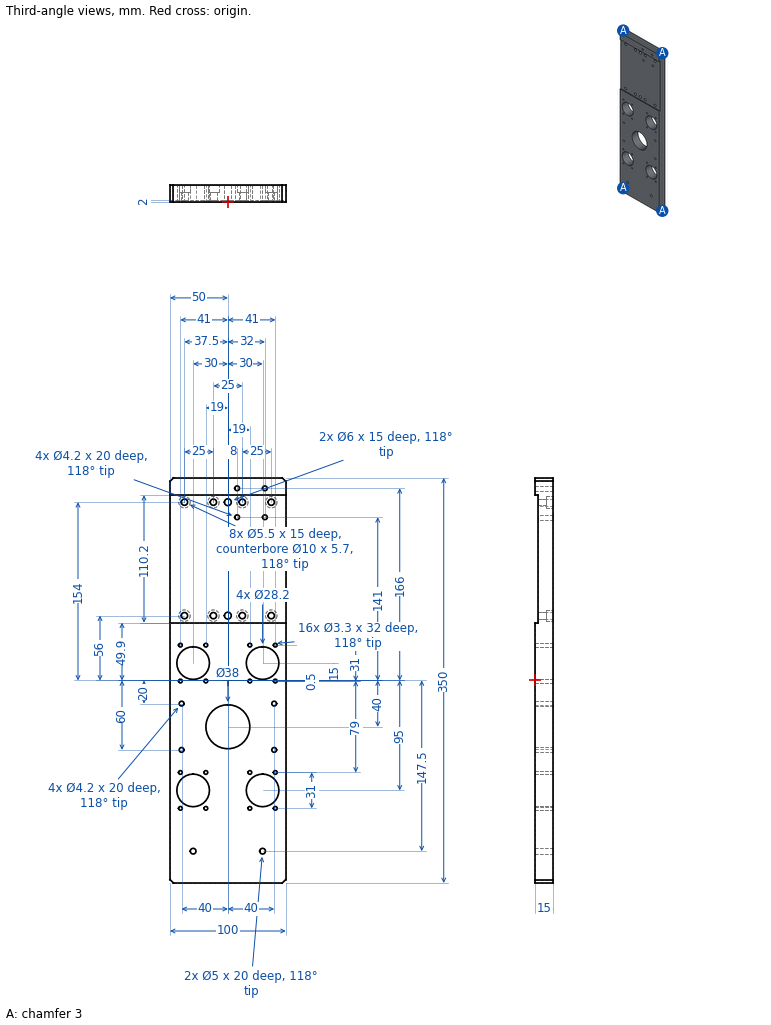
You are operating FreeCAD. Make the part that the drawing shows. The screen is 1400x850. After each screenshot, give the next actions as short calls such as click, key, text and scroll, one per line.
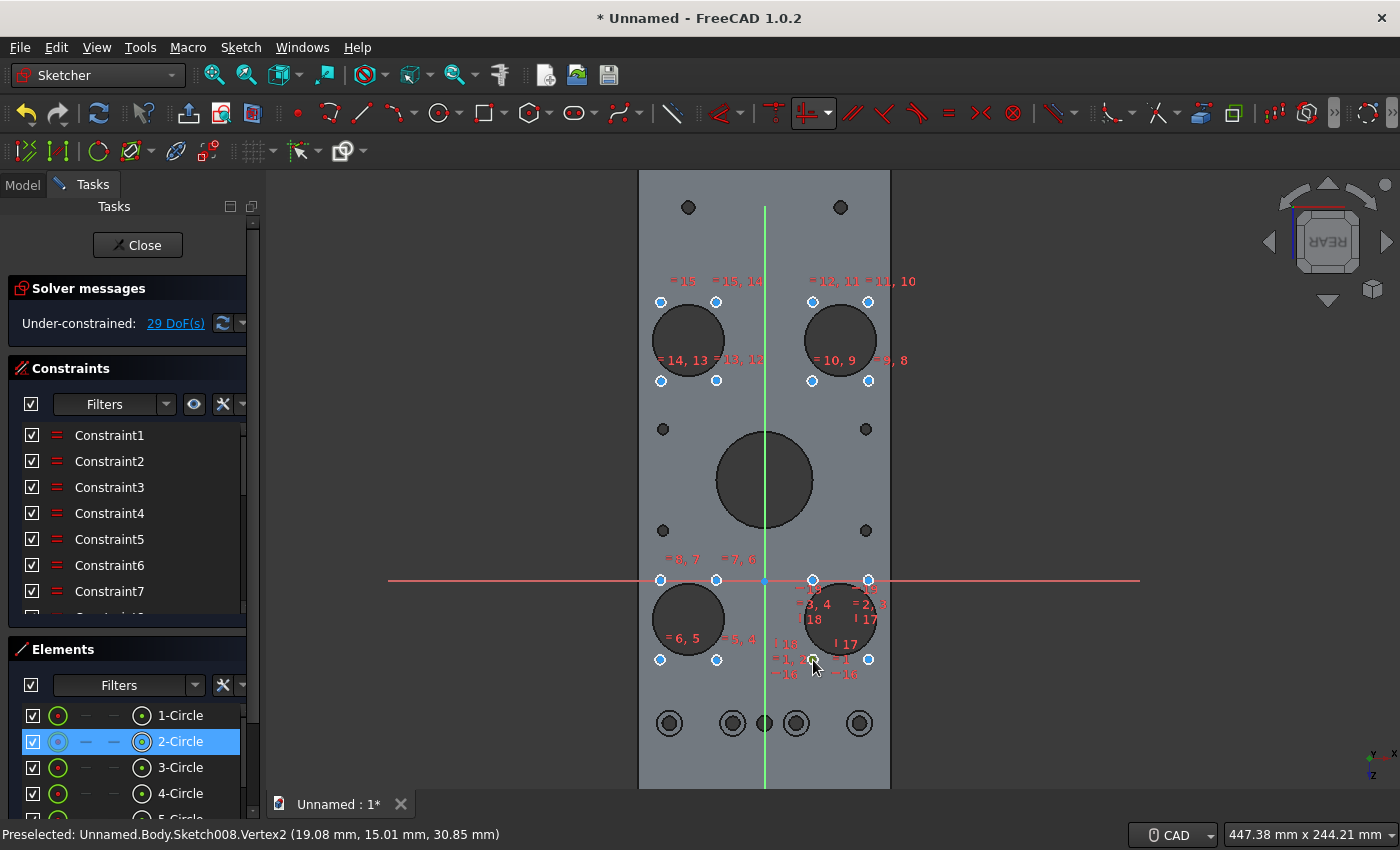
click(717, 660)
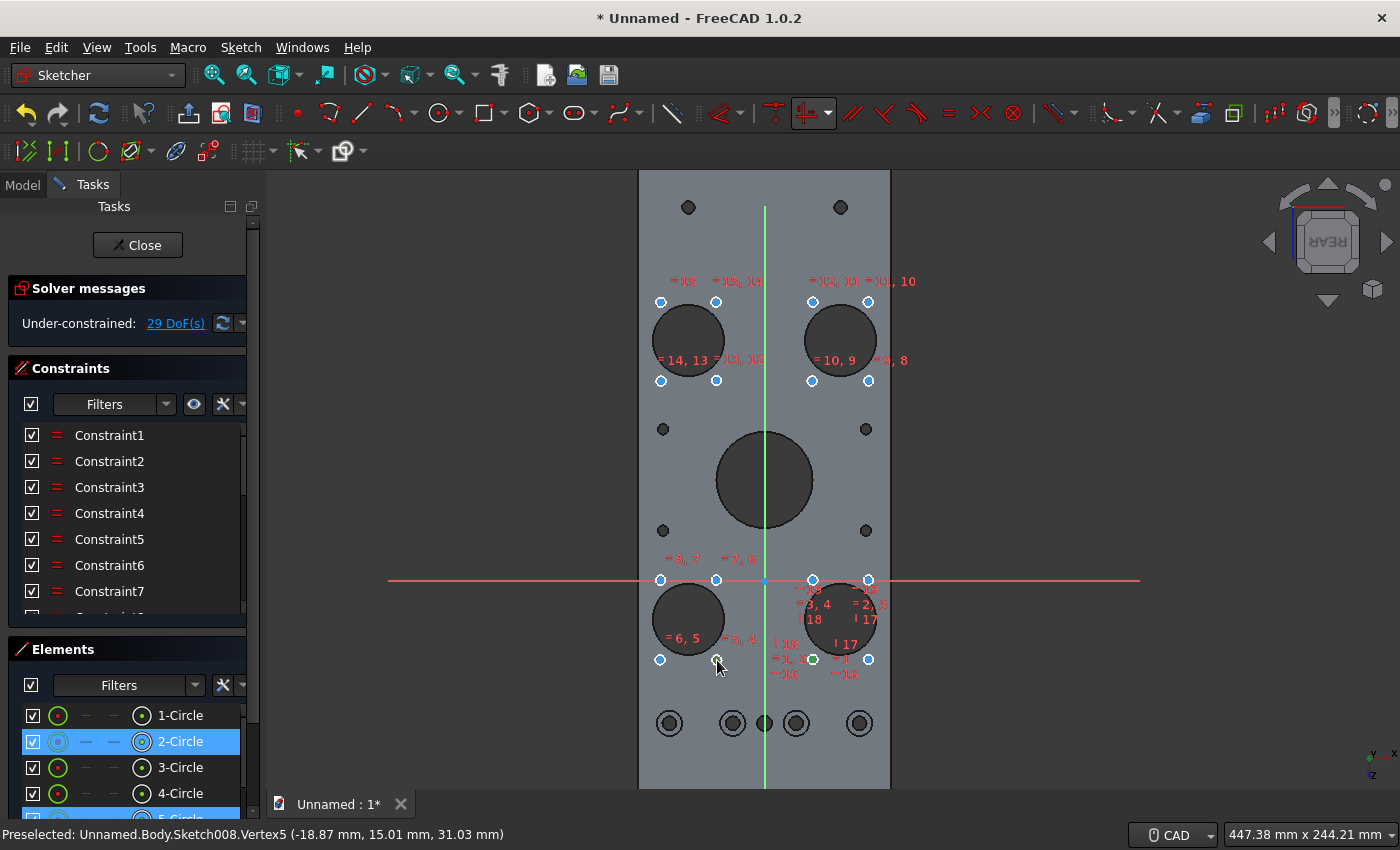
key(h)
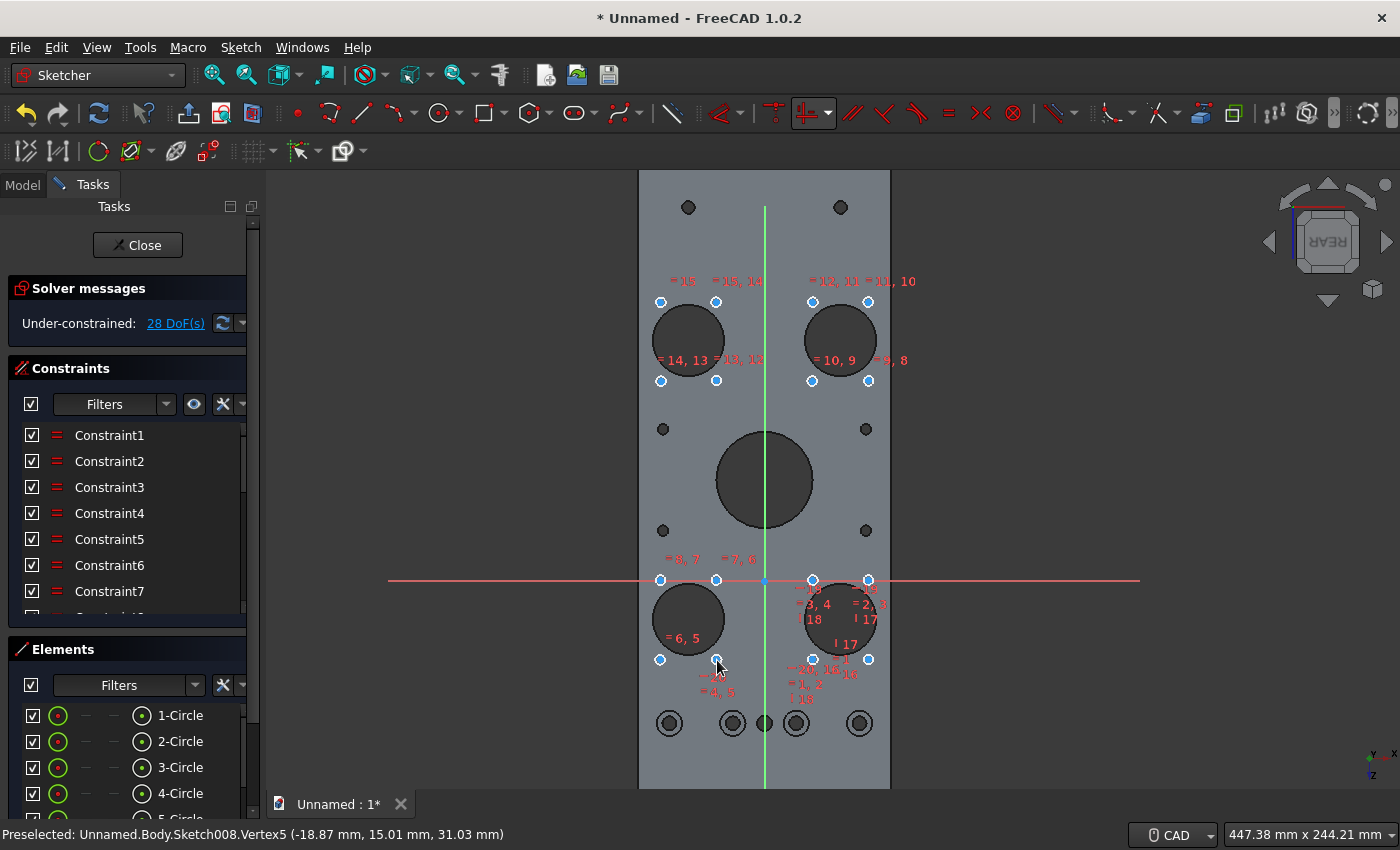
click(717, 660)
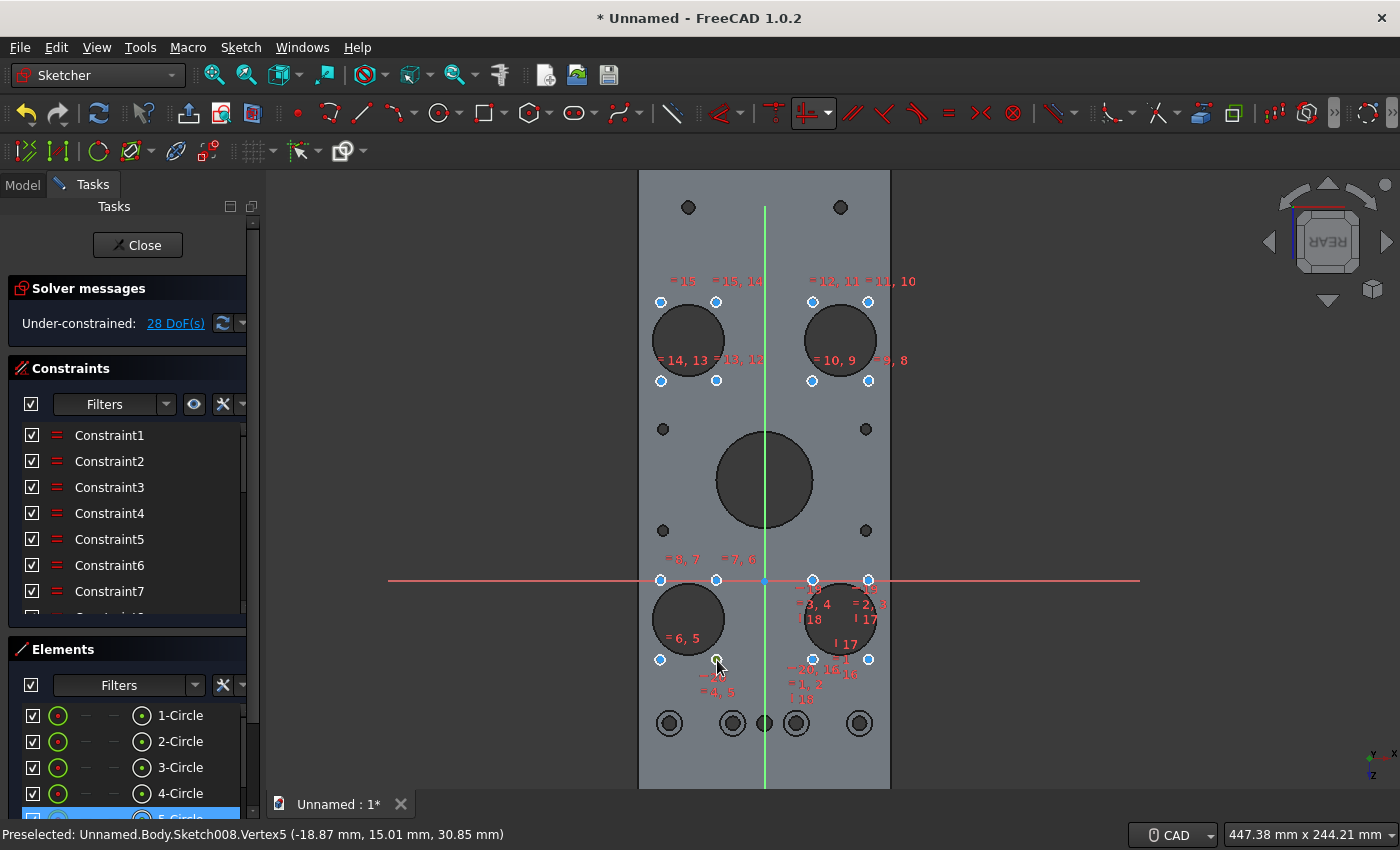
click(660, 660)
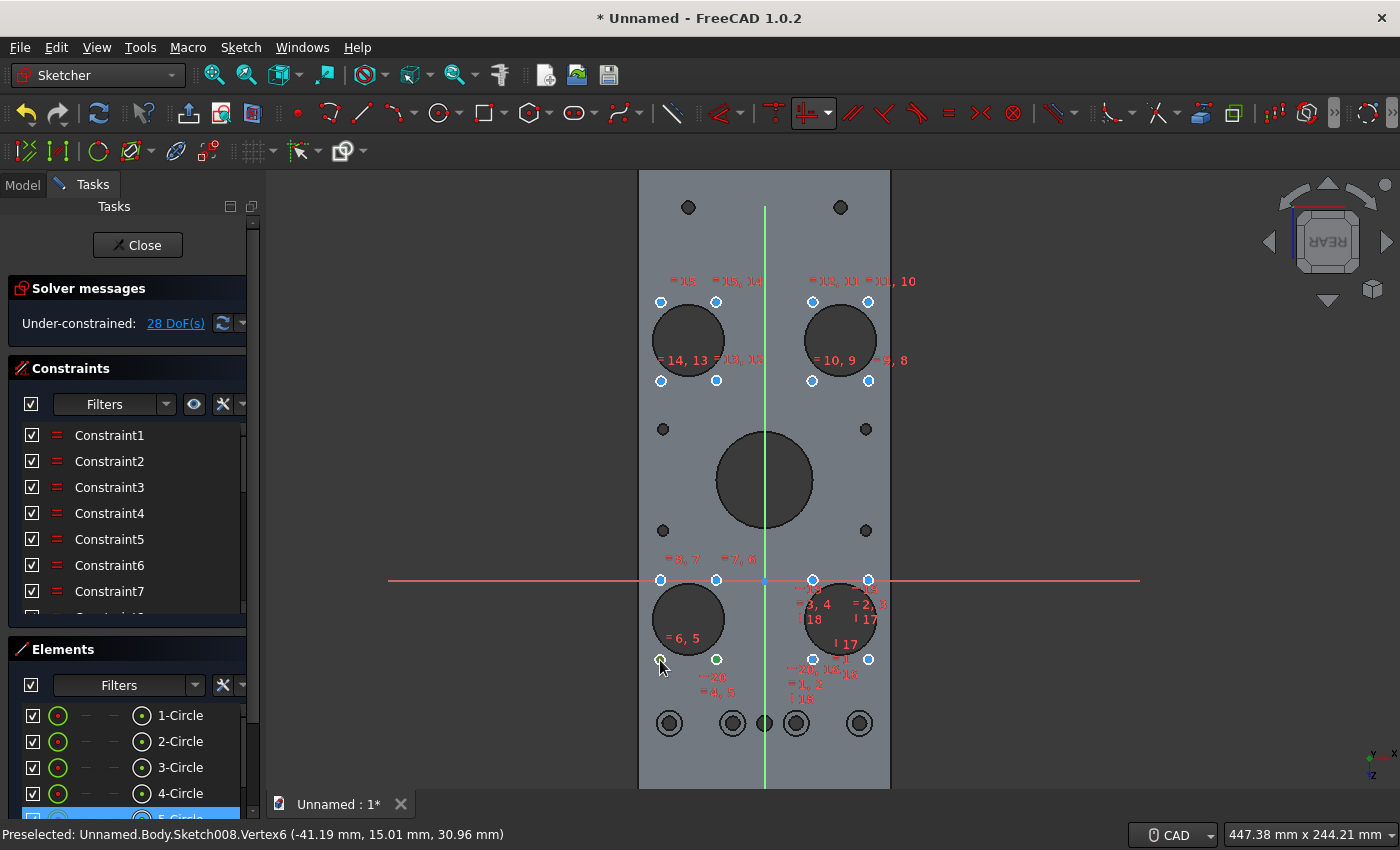
click(830, 114)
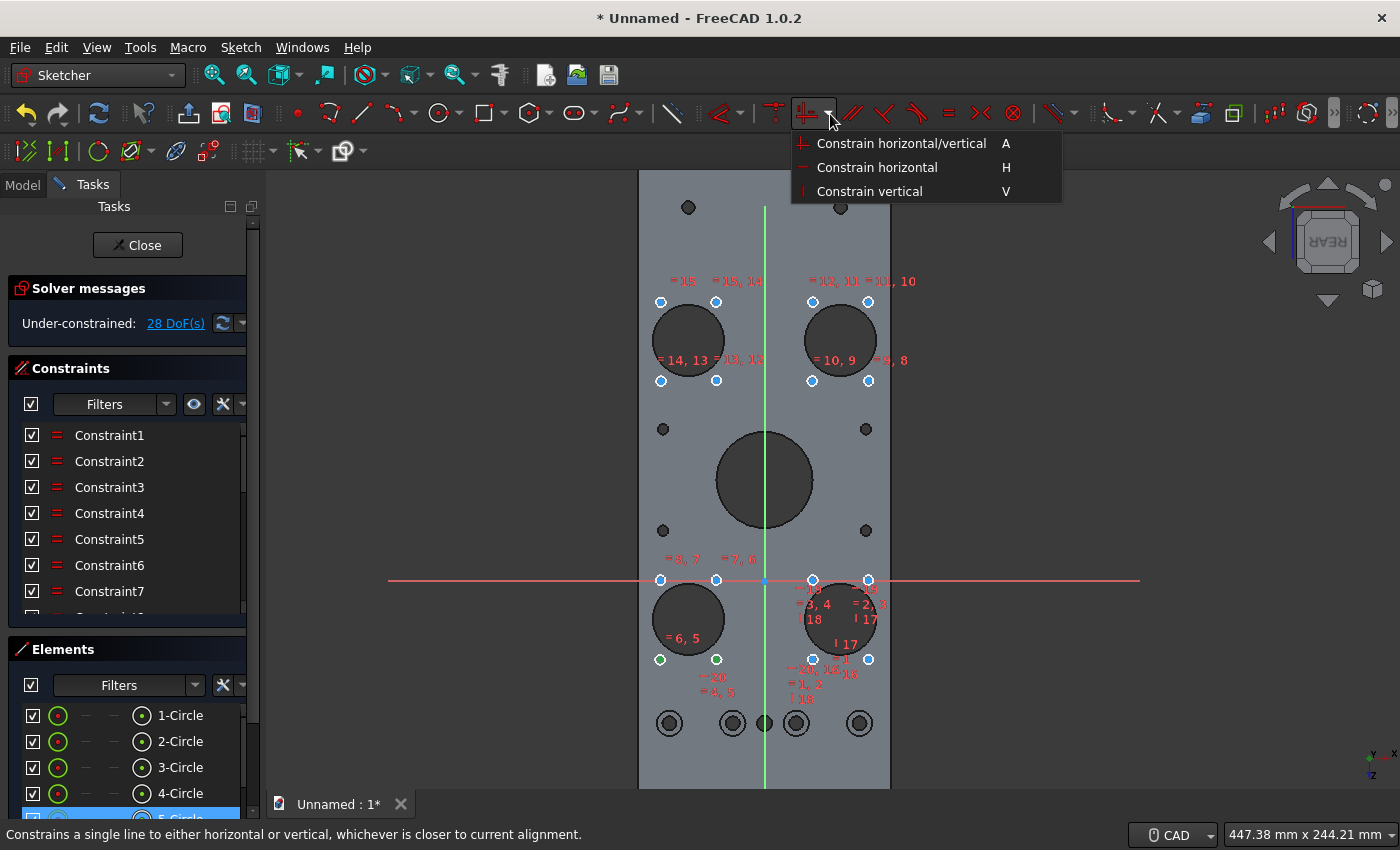
click(927, 167)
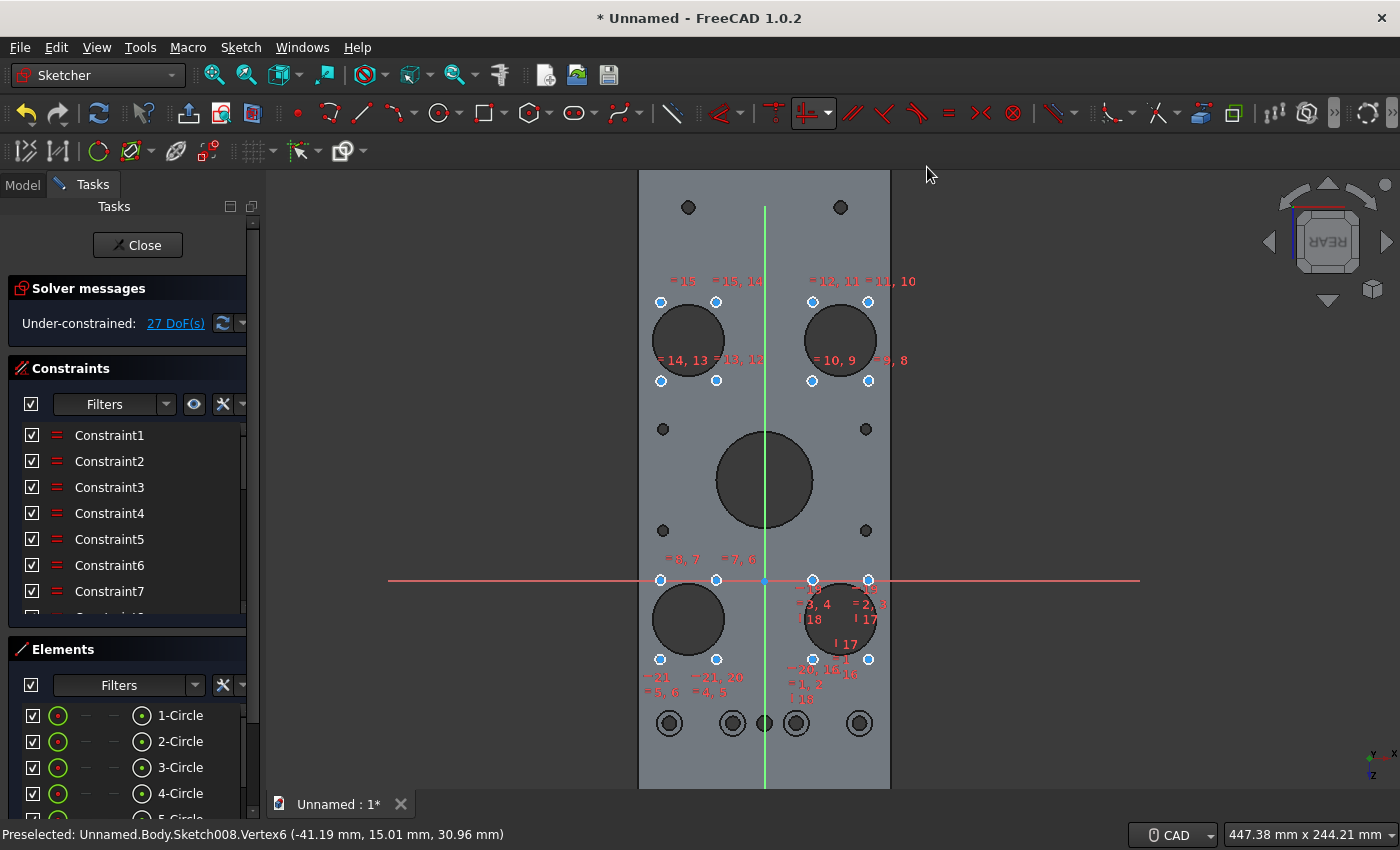
click(717, 660)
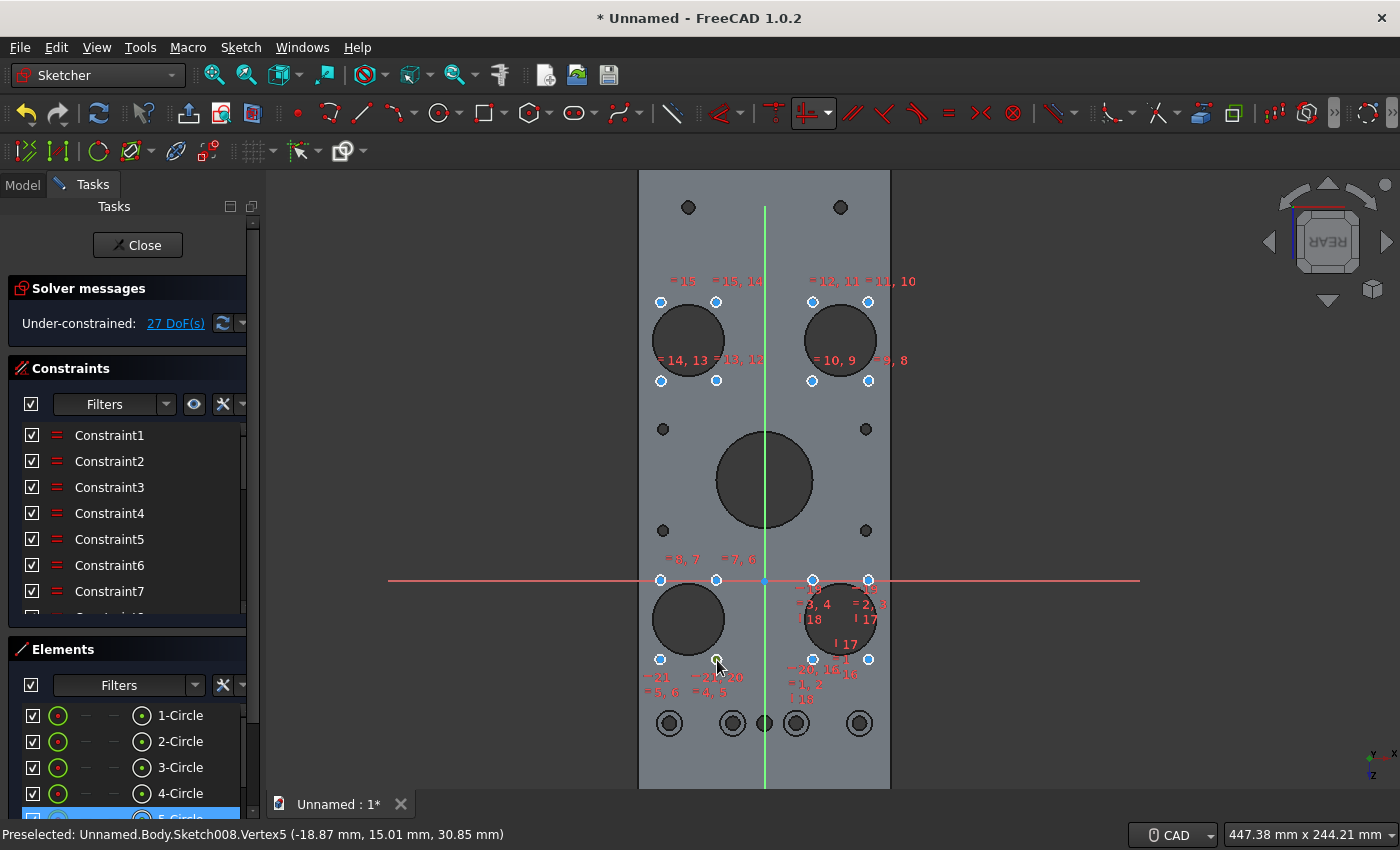
click(716, 580)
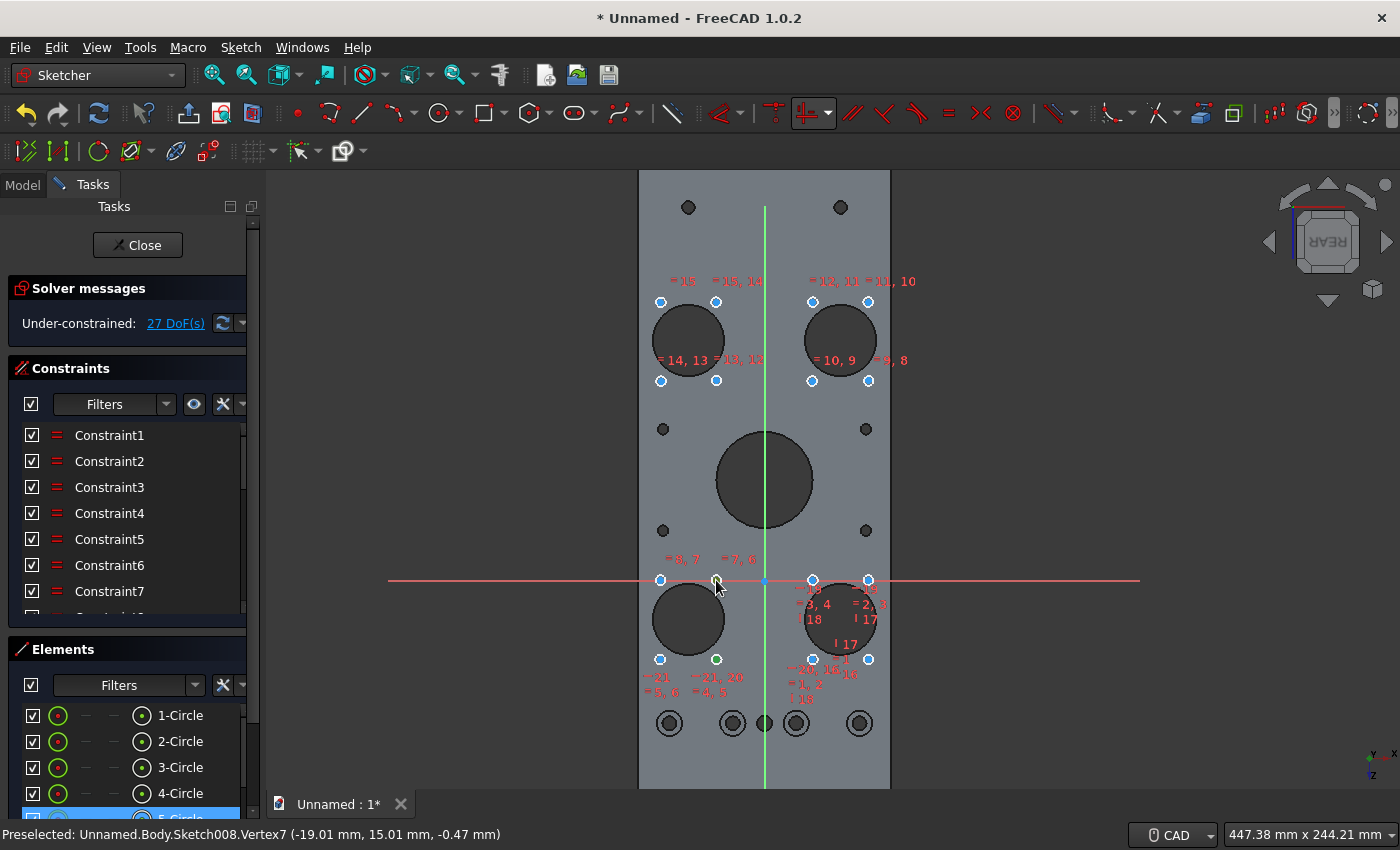
click(830, 114)